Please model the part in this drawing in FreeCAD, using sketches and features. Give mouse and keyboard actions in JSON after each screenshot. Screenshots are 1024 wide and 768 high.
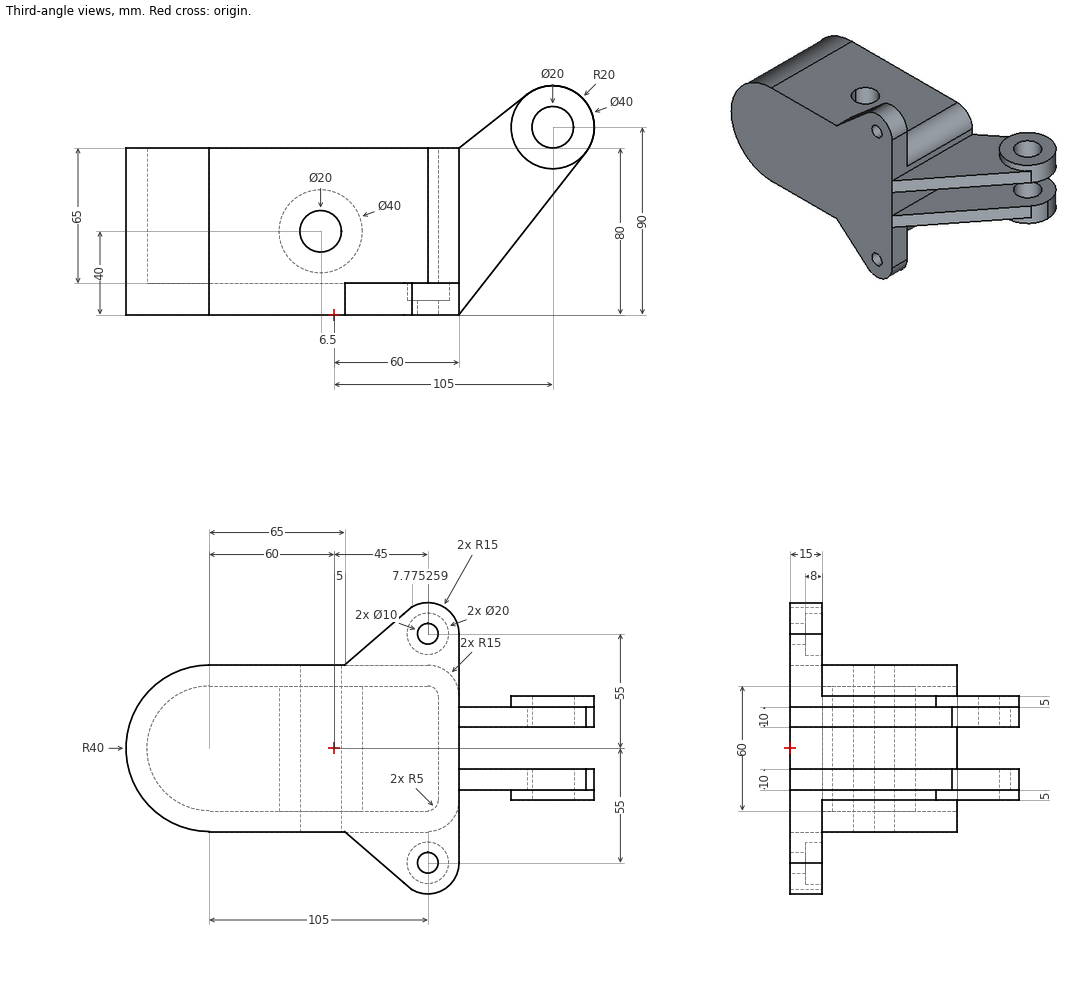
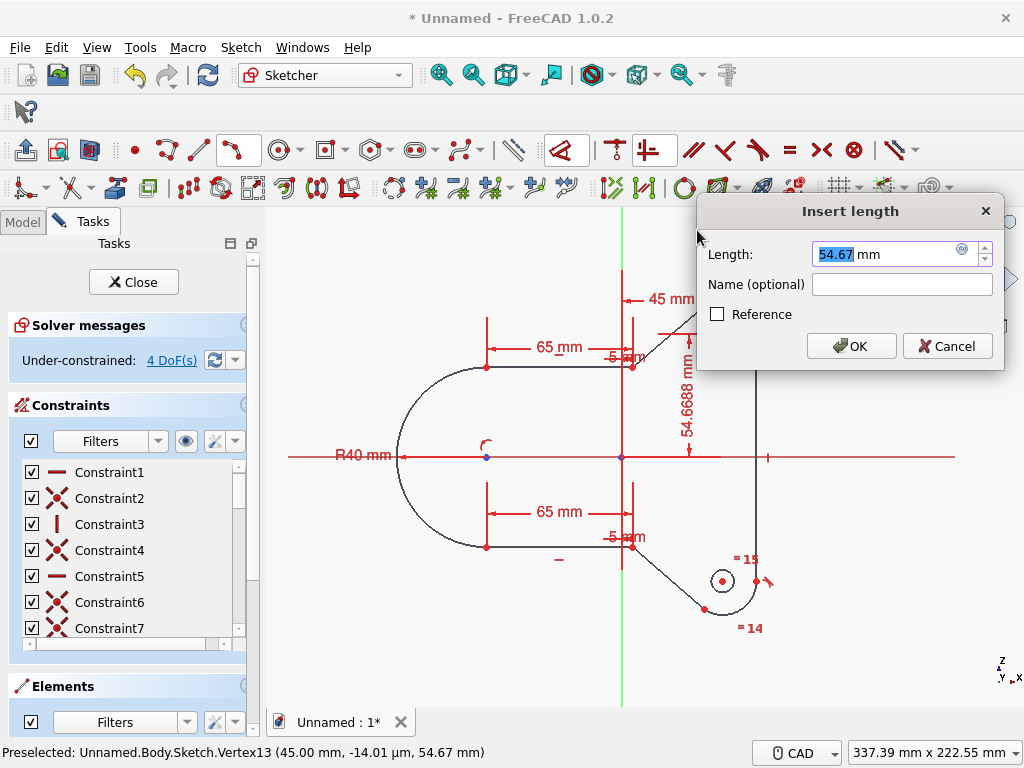
{"action": "type", "text": "55"}
{"action": "key", "text": "Return"}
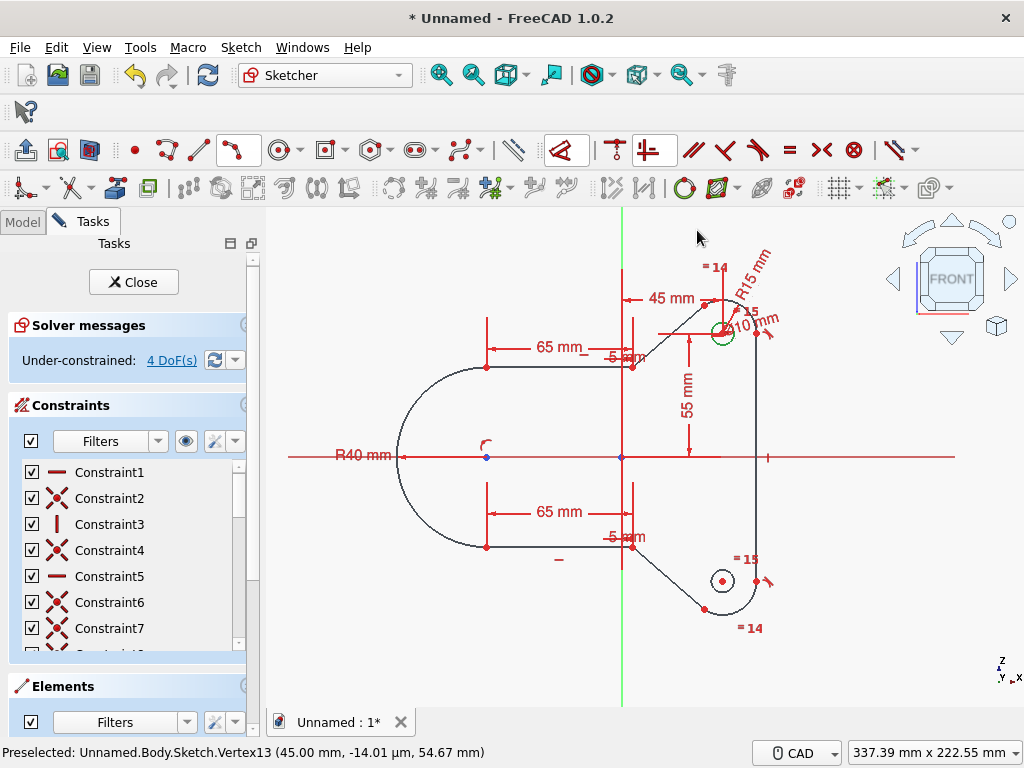
{"action": "left_click", "coordinate": [723, 581]}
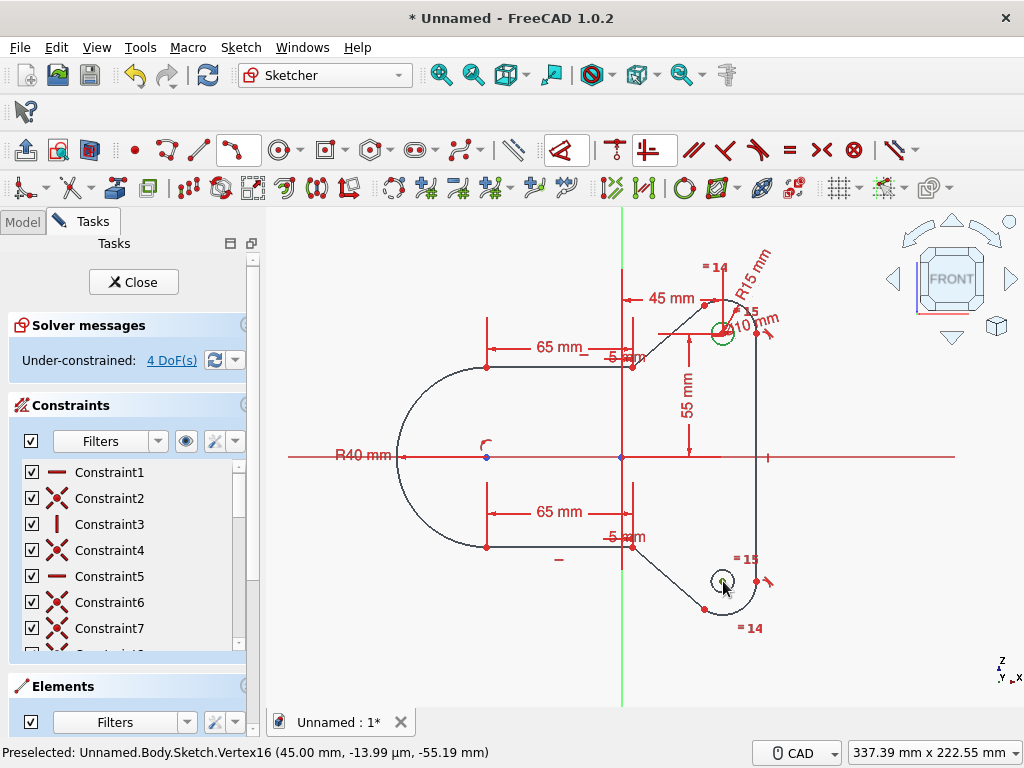
{"action": "key", "text": "i"}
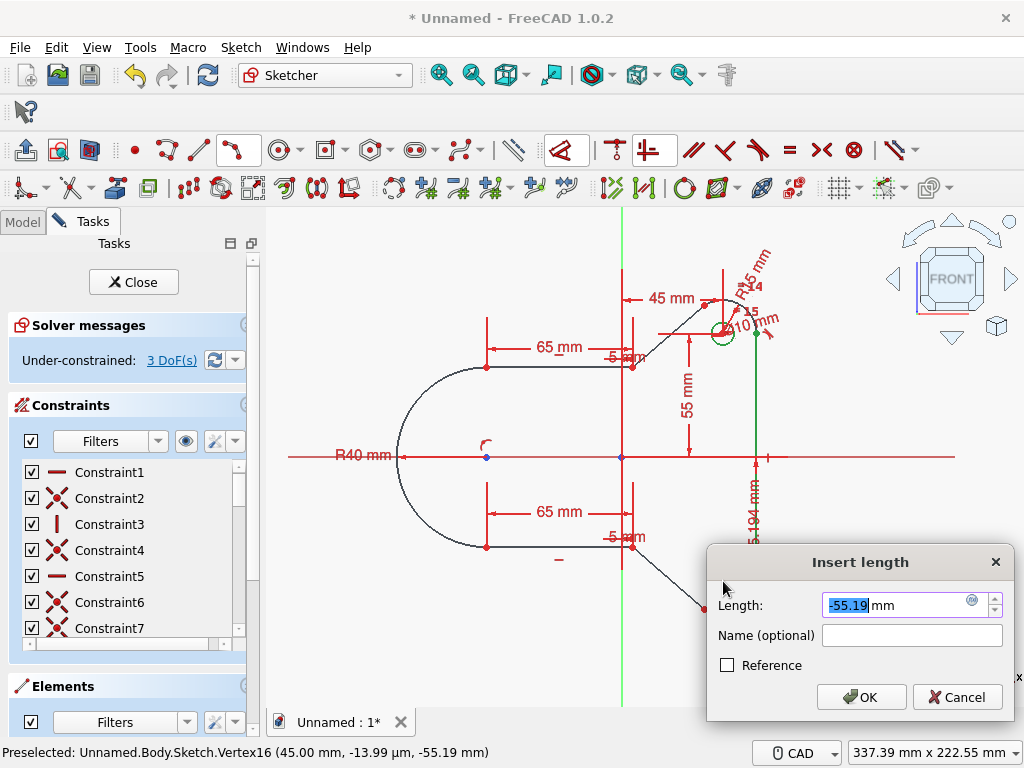
{"action": "type", "text": "-55"}
{"action": "key", "text": "Return"}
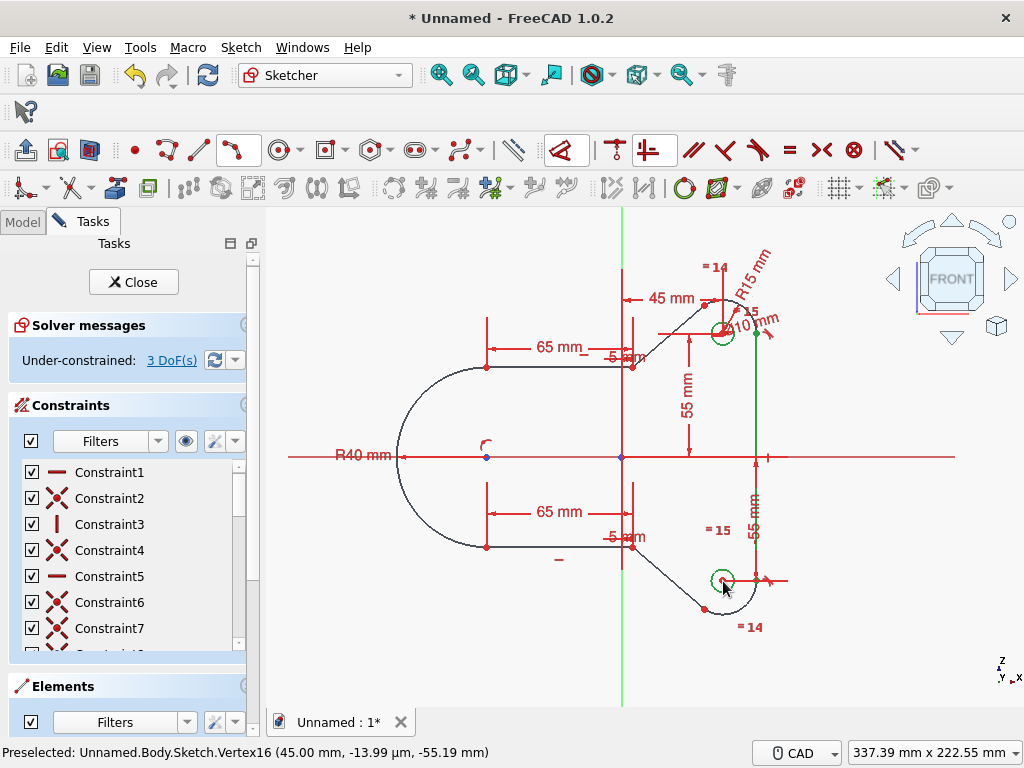
{"action": "left_click", "coordinate": [487, 457]}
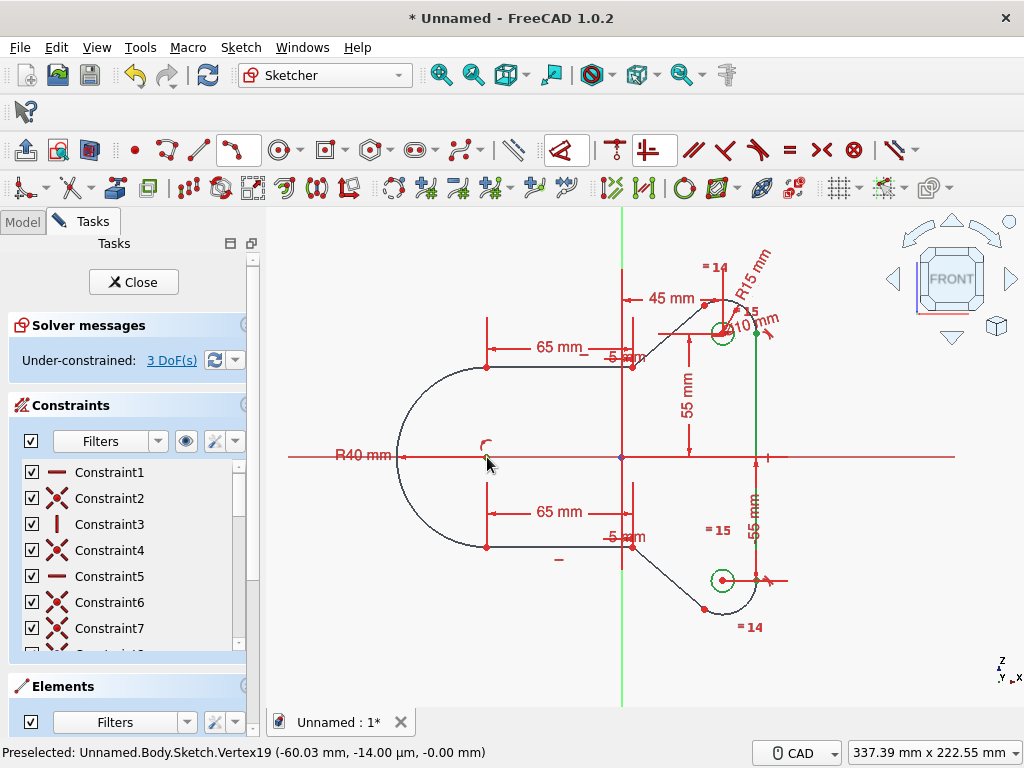
{"action": "key", "text": "l"}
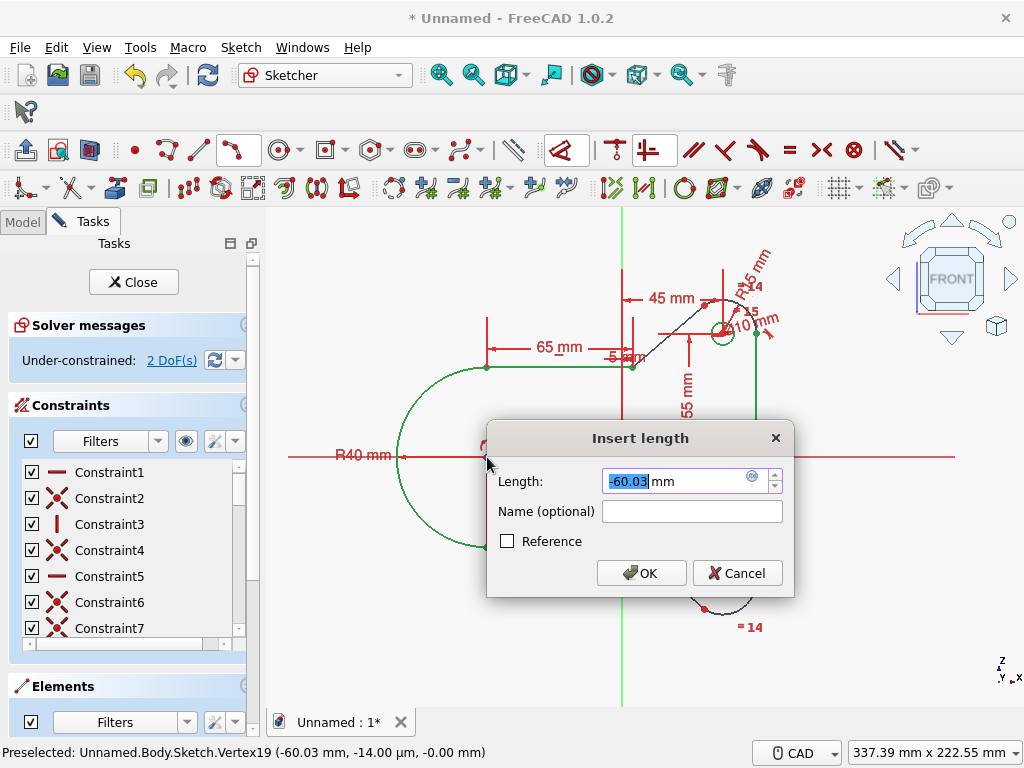
{"action": "type", "text": "-60"}
{"action": "key", "text": "Return"}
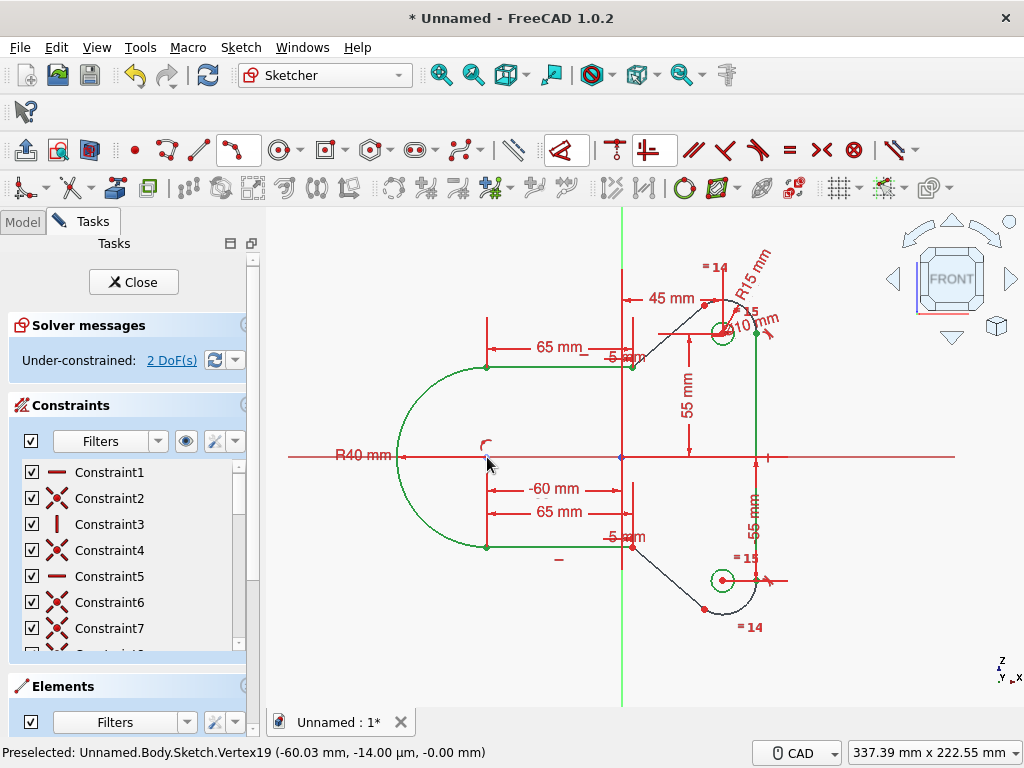
{"action": "scroll", "coordinate": [705, 305], "scroll_direction": "up", "scroll_amount": 5}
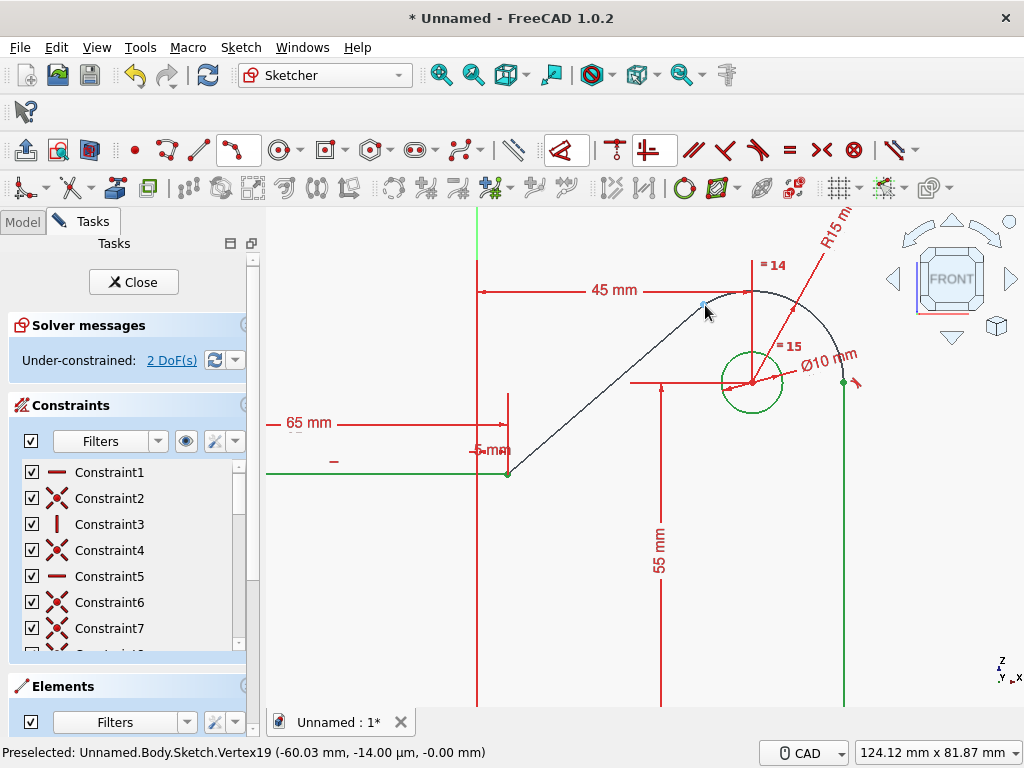
{"action": "left_click", "coordinate": [704, 305]}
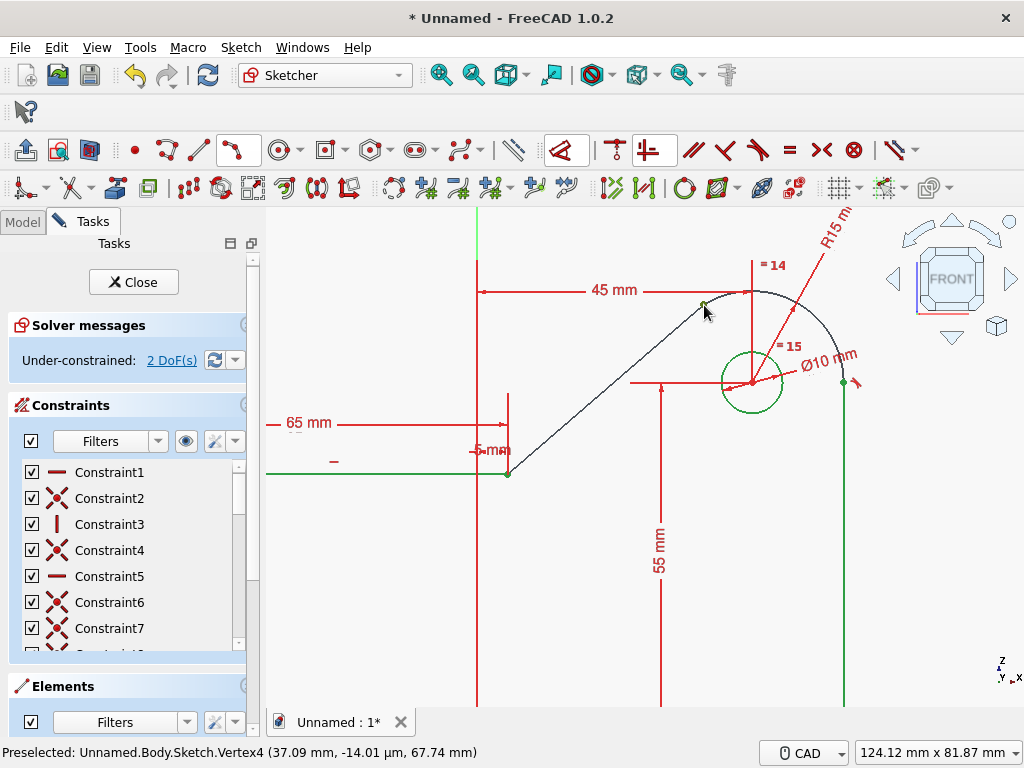
{"action": "left_click", "coordinate": [752, 383]}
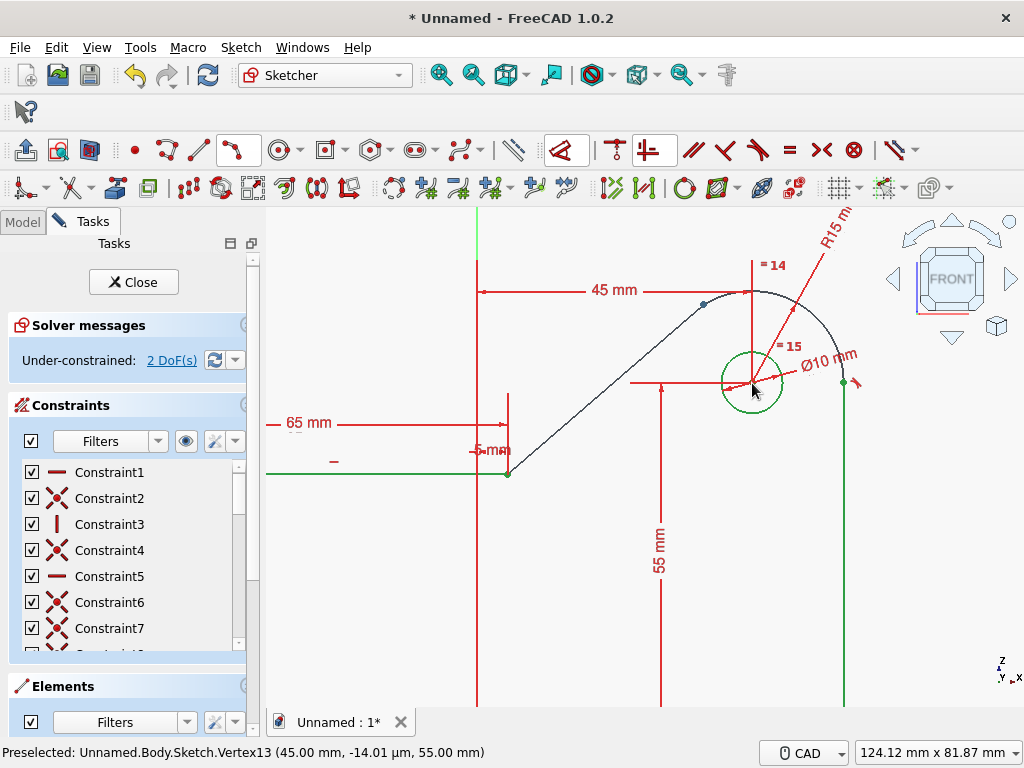
{"action": "left_click", "coordinate": [584, 150]}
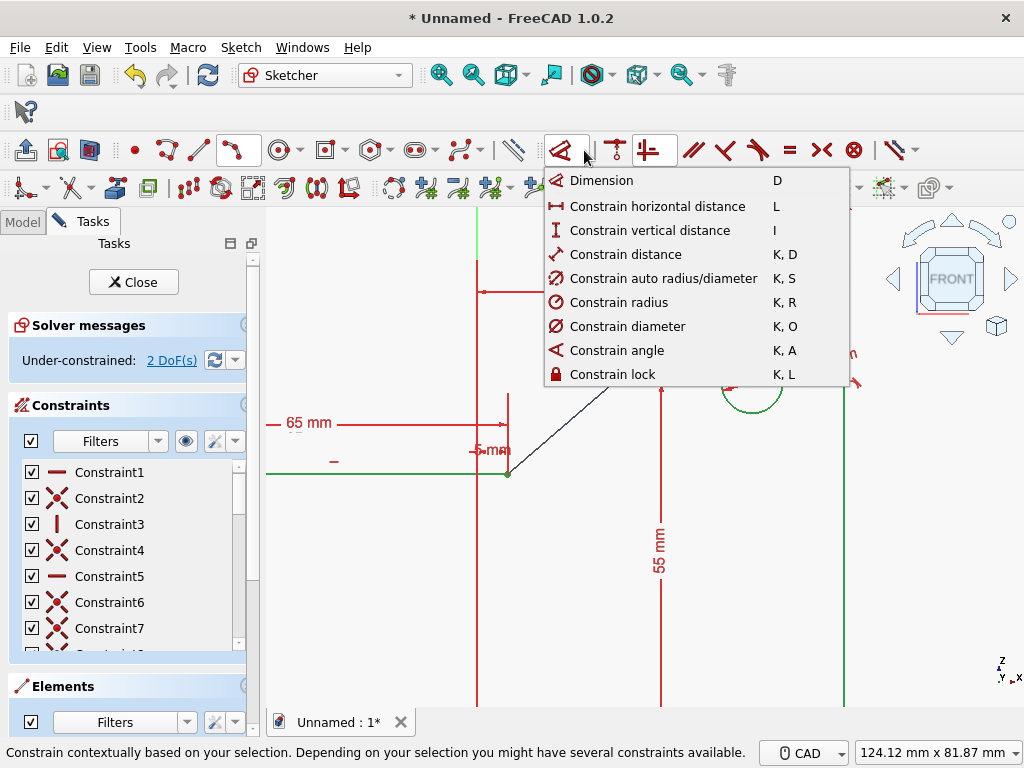
{"action": "left_click", "coordinate": [697, 206]}